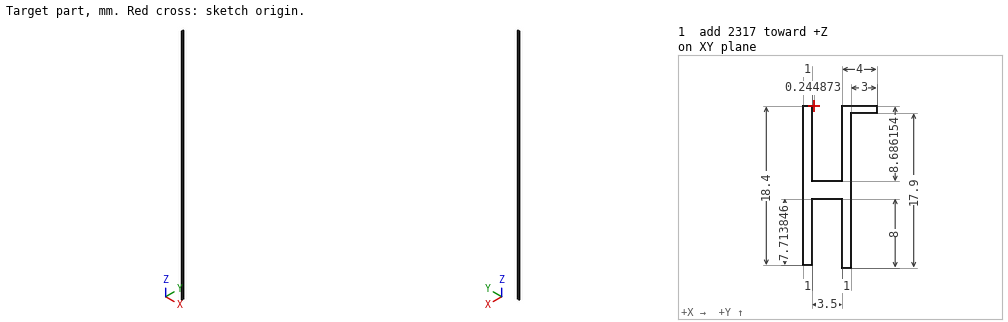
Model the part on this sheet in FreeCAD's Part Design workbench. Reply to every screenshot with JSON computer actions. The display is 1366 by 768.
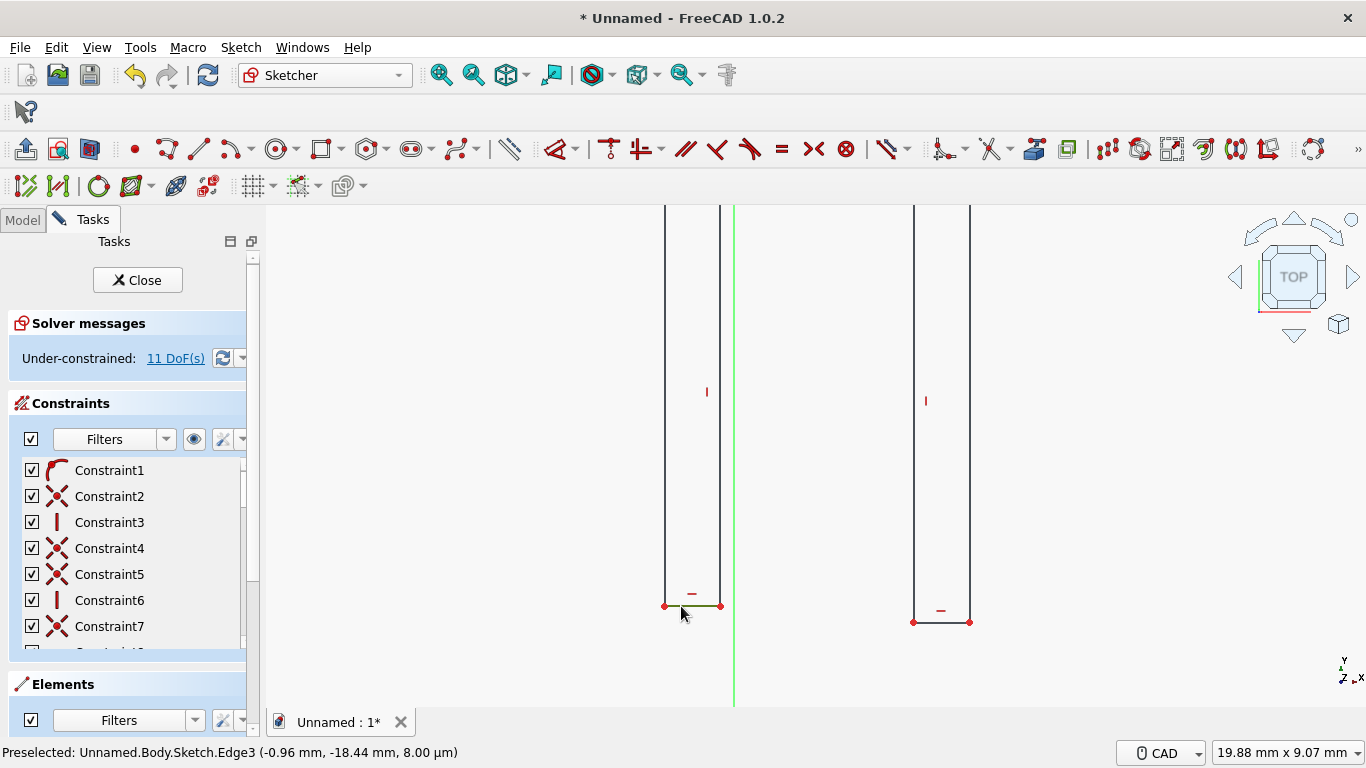
{"action": "key", "text": "l"}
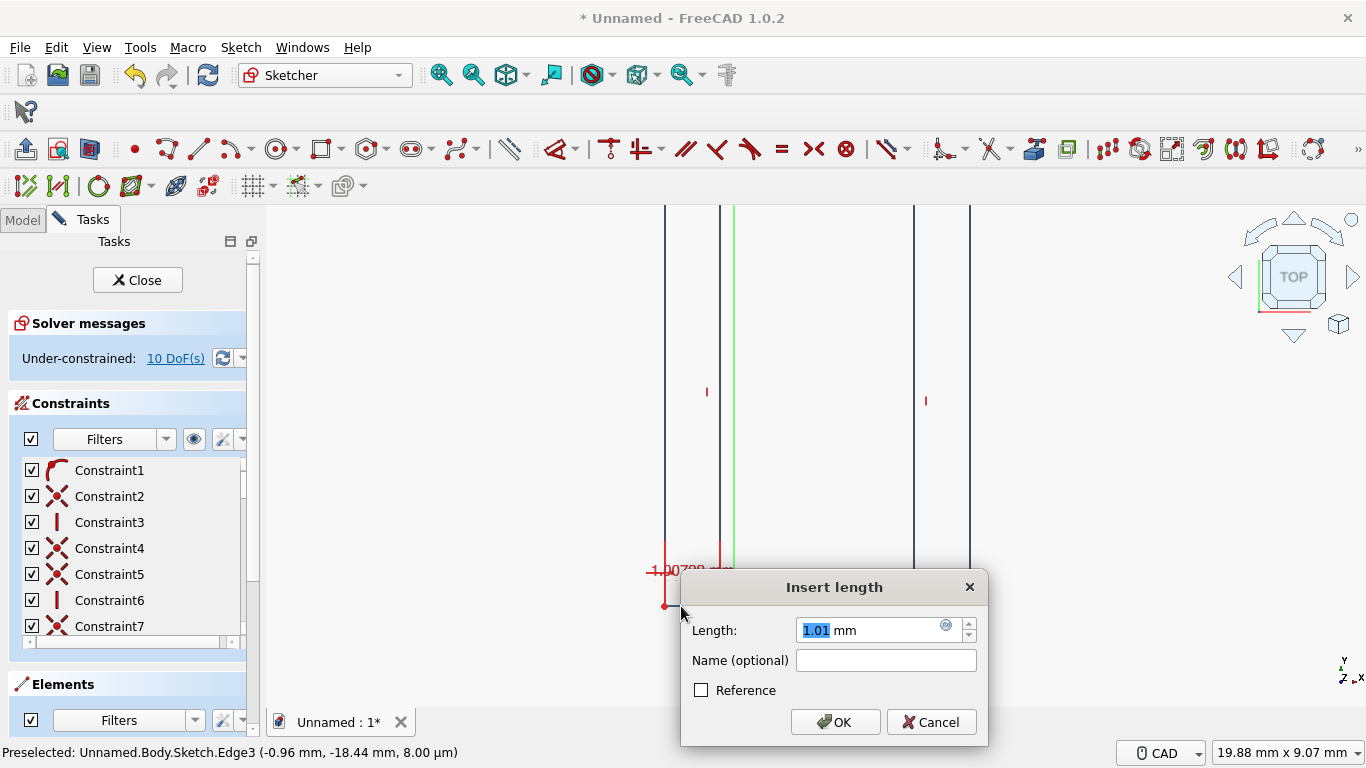
{"action": "type", "text": "1"}
{"action": "key", "text": "Return"}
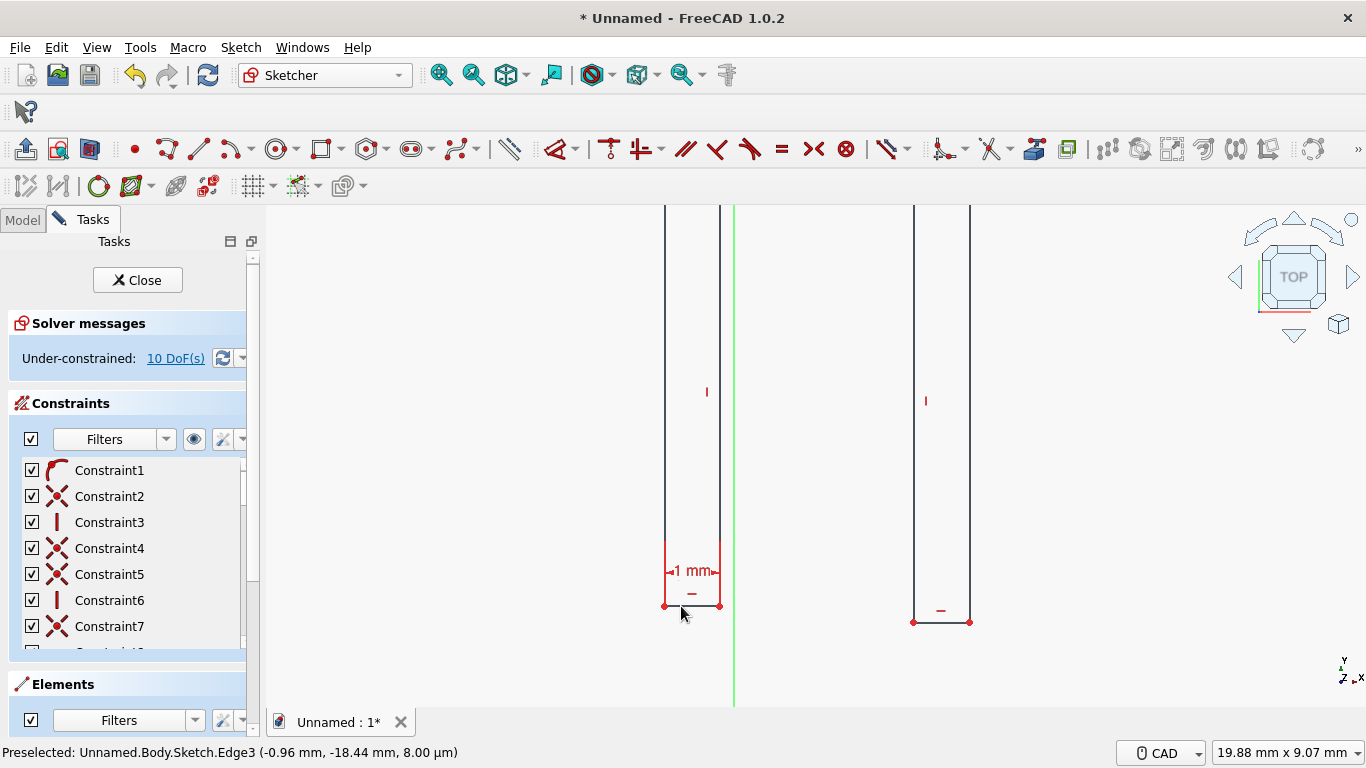
{"action": "left_click", "coordinate": [914, 311]}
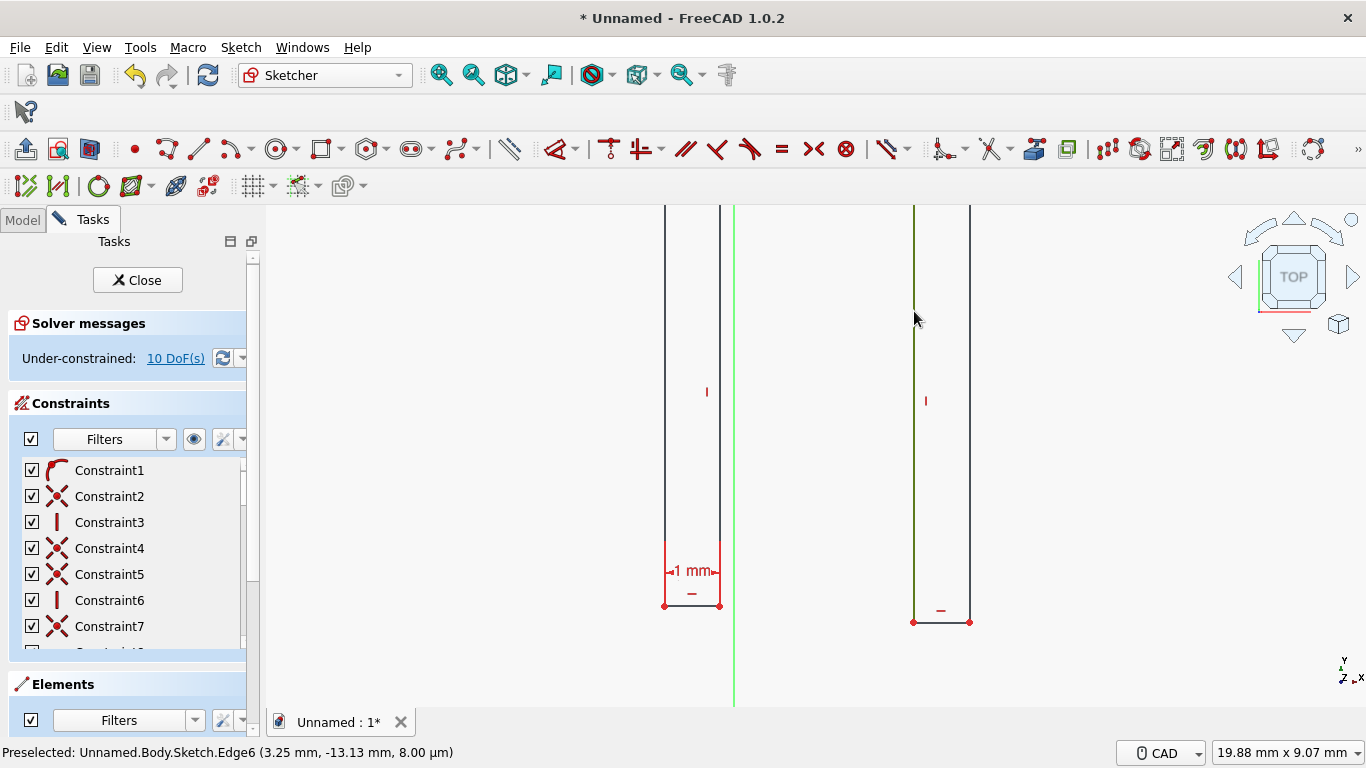
{"action": "left_click", "coordinate": [578, 150]}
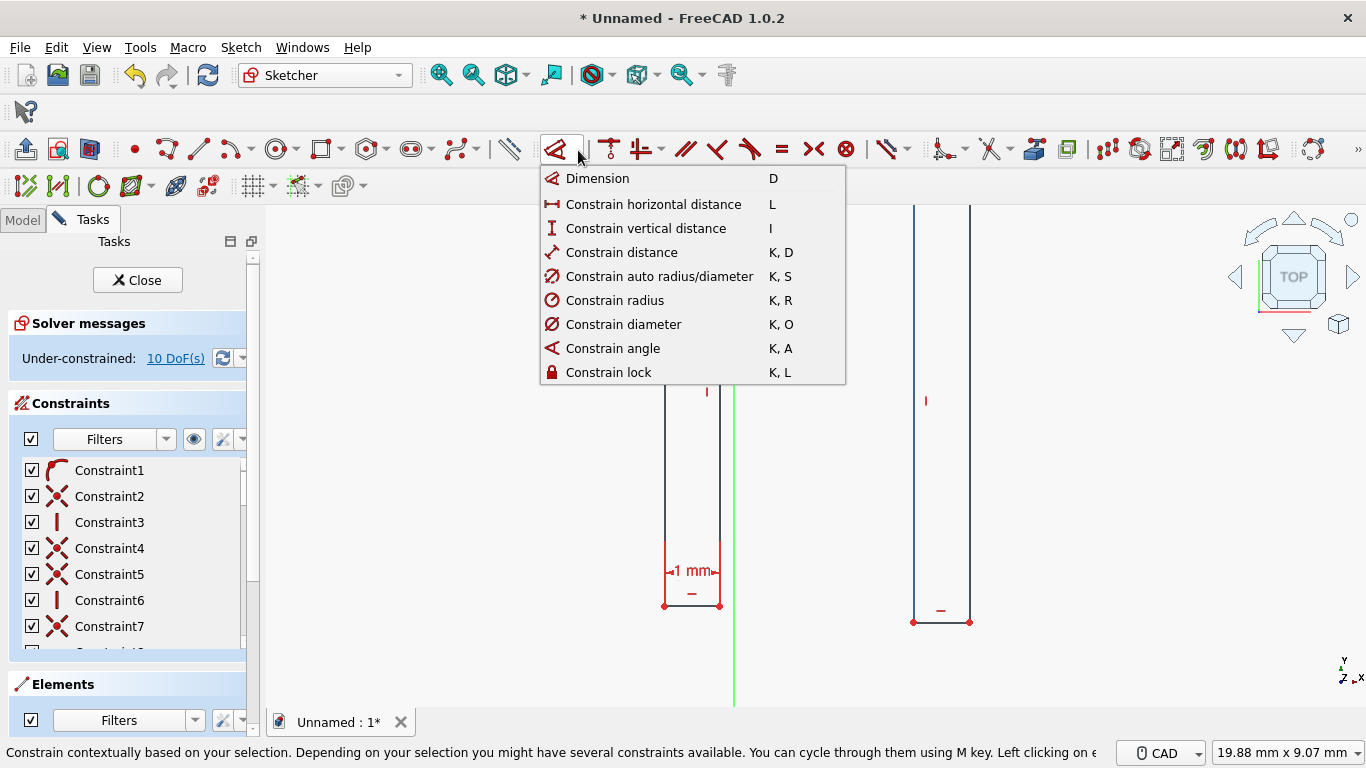
{"action": "left_click", "coordinate": [693, 228]}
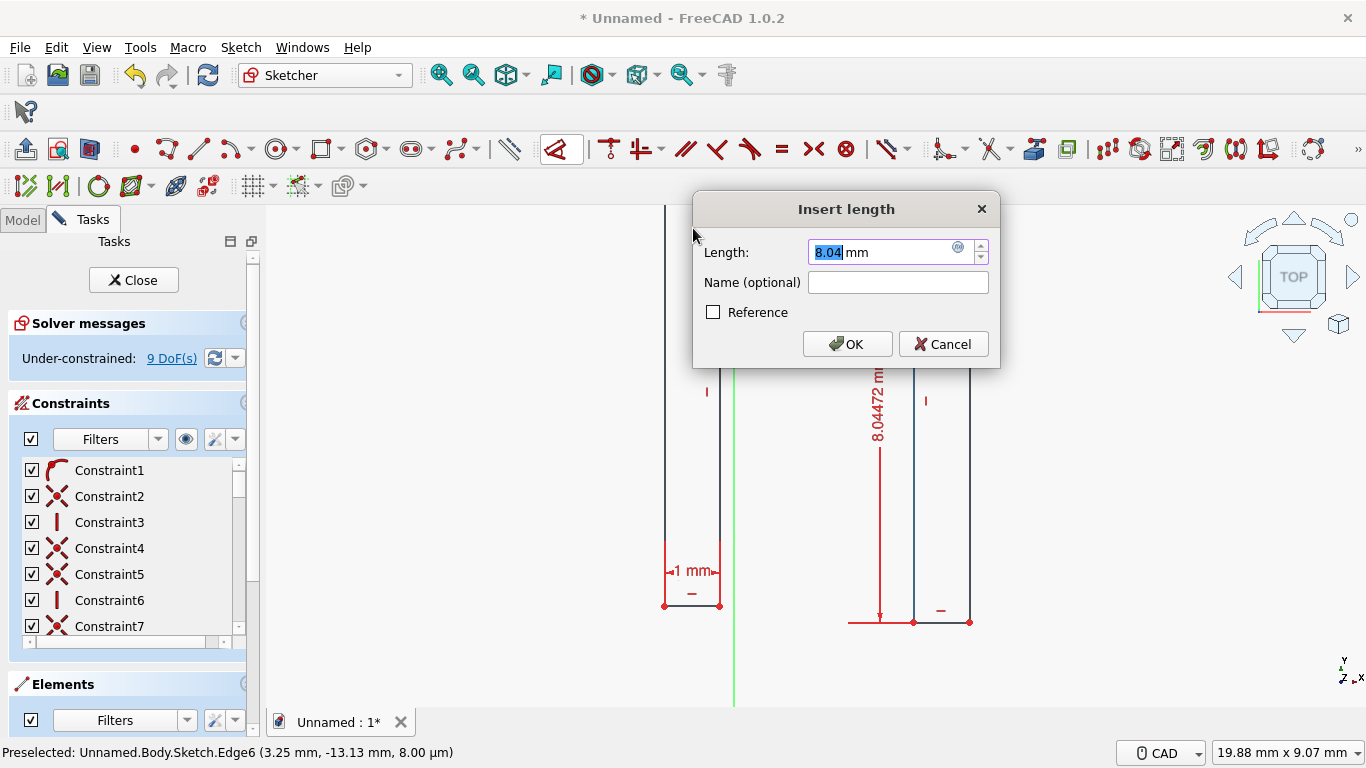
{"action": "type", "text": "8"}
{"action": "key", "text": "Return"}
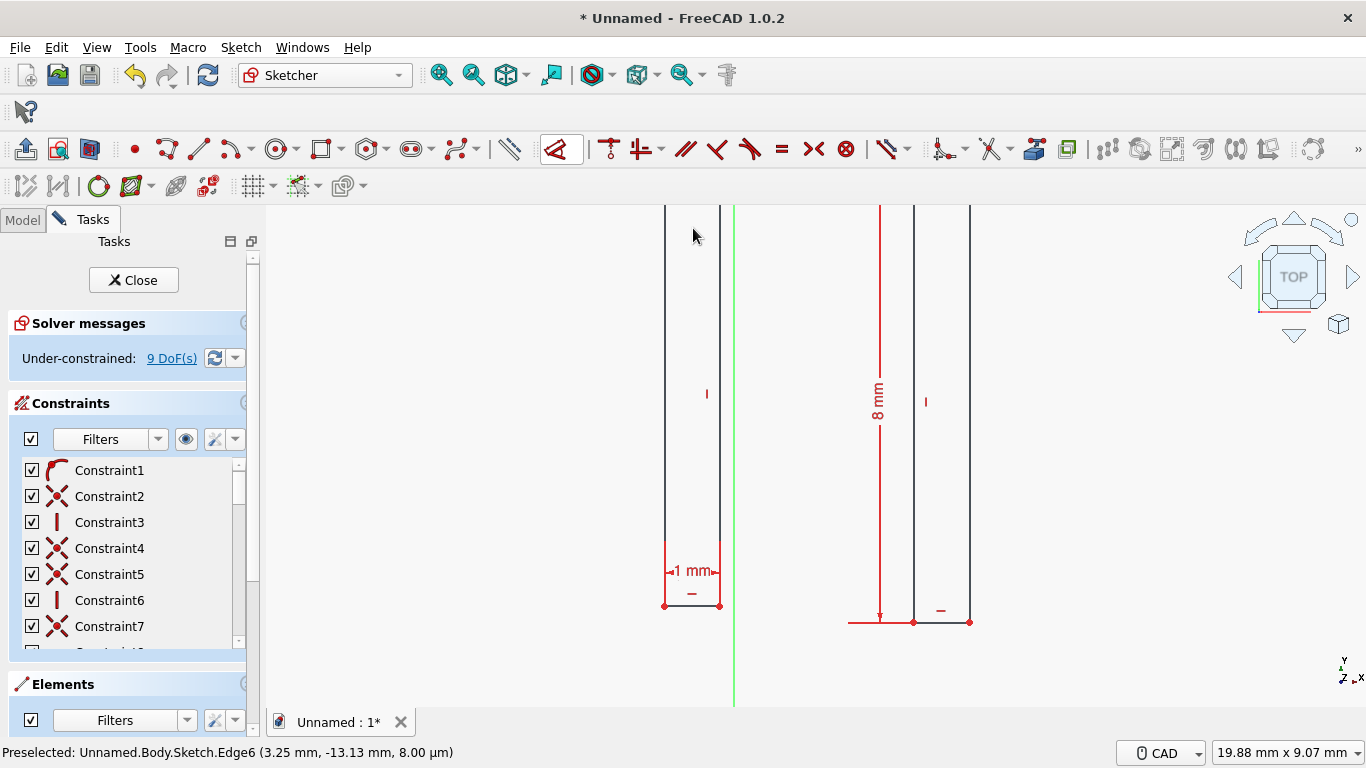
{"action": "left_click", "coordinate": [930, 623]}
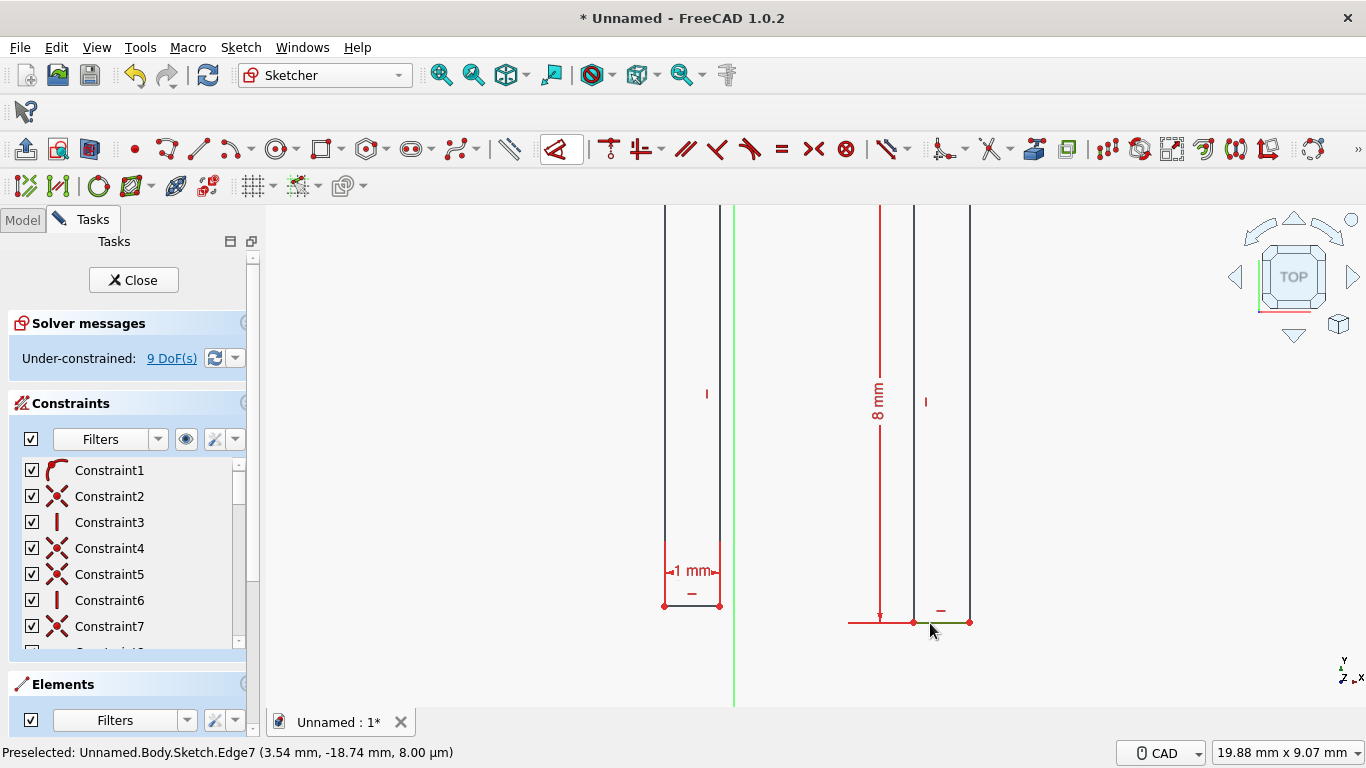
{"action": "key", "text": "l"}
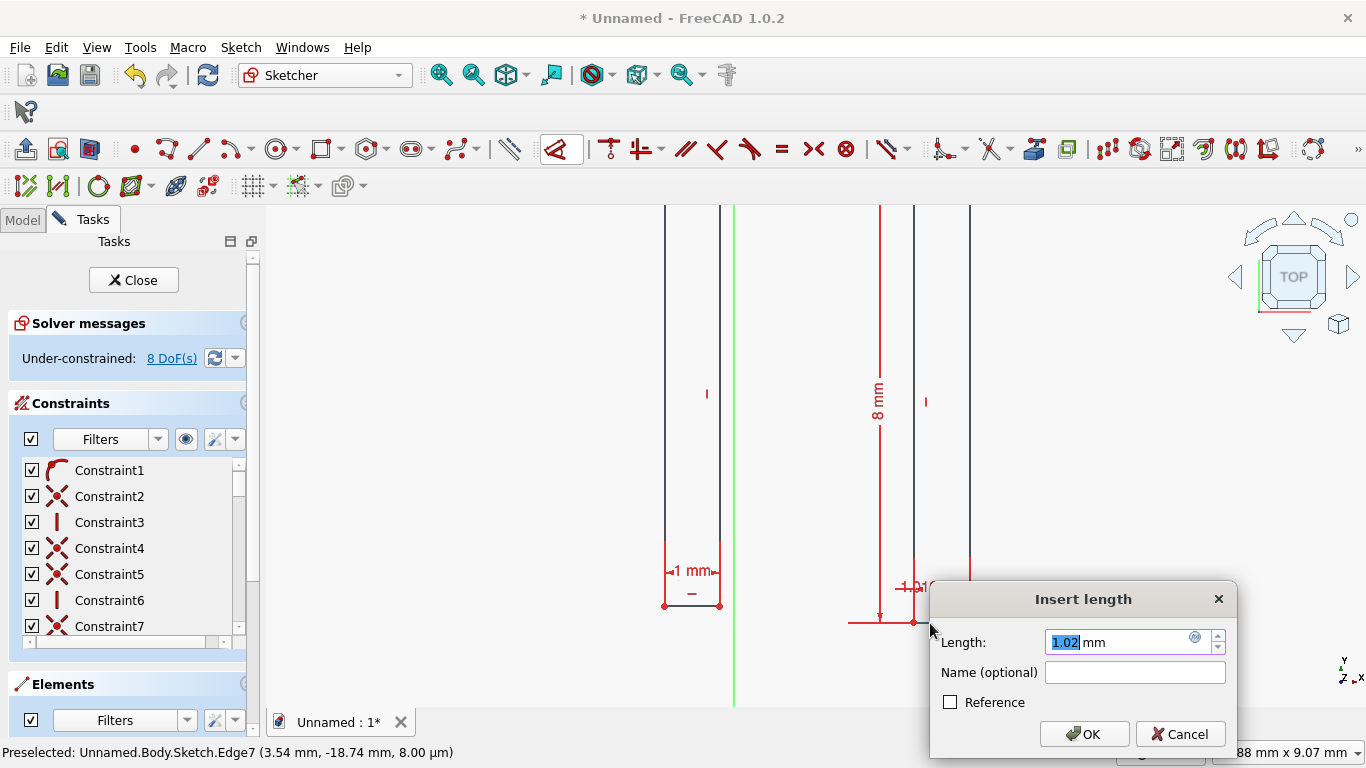
{"action": "type", "text": "1"}
{"action": "key", "text": "Return"}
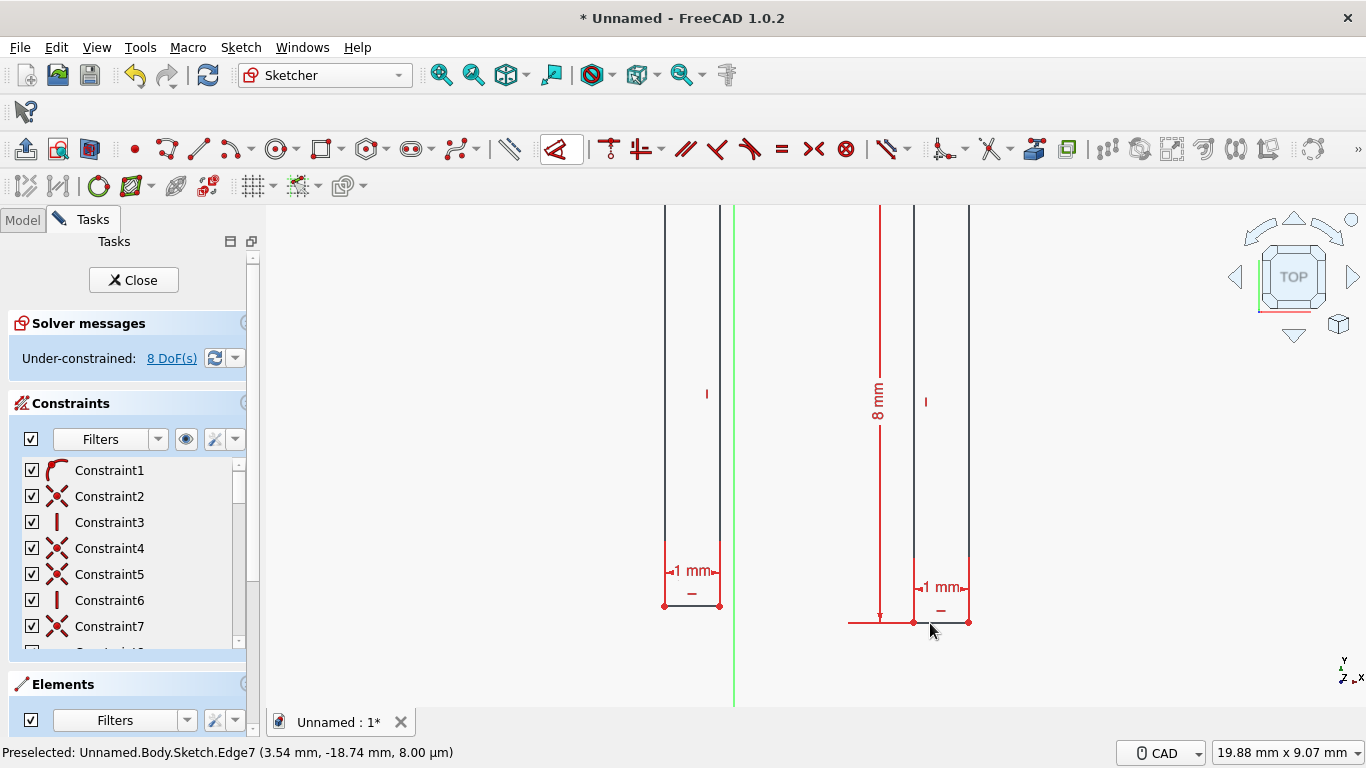
{"action": "scroll", "coordinate": [682, 608], "scroll_direction": "down", "scroll_amount": 6}